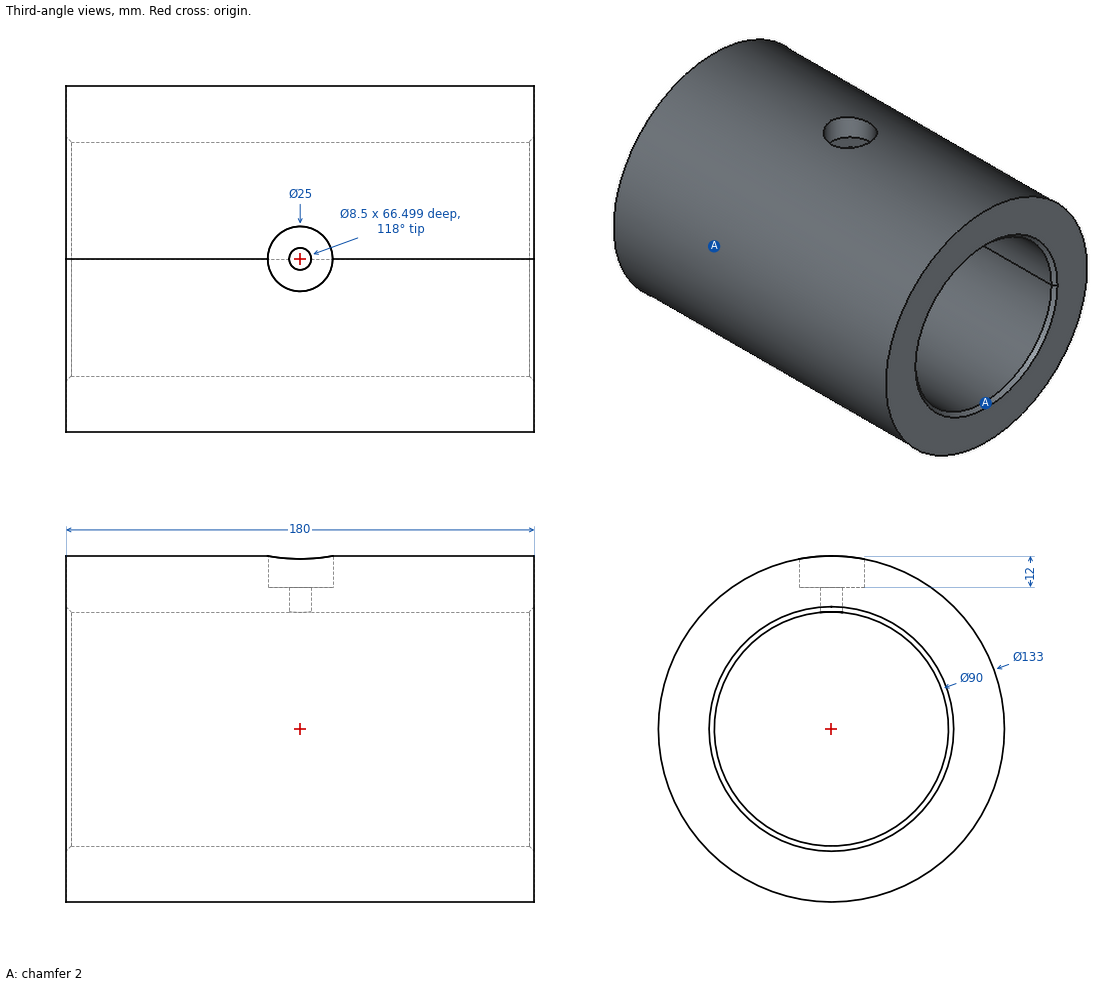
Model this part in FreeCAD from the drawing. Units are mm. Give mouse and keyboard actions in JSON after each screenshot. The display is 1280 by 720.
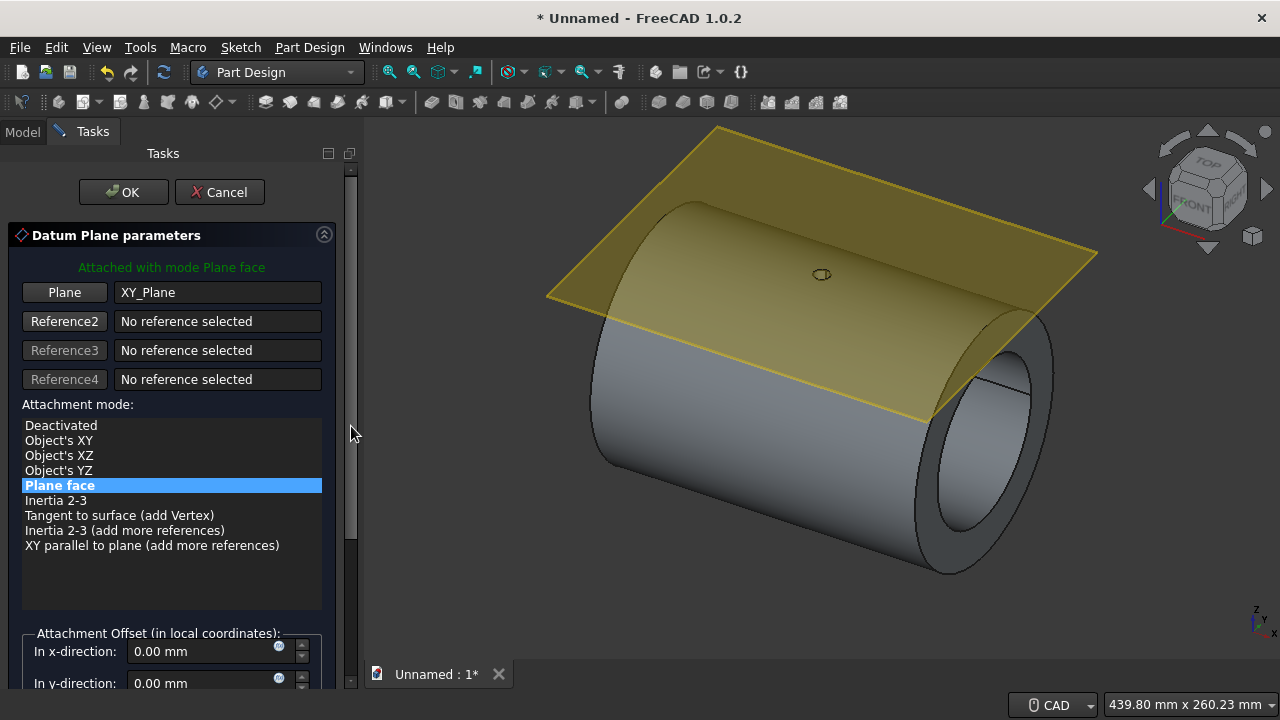
{"action": "left_click", "coordinate": [124, 192]}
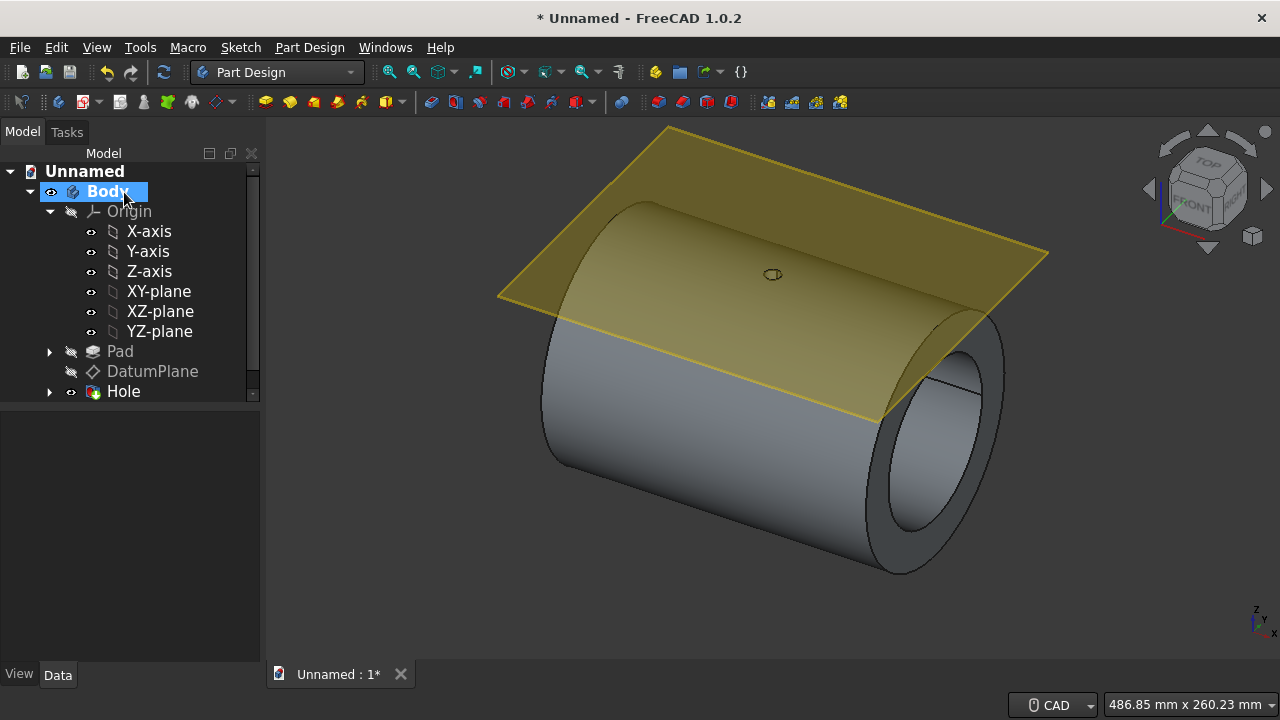
{"action": "scroll", "coordinate": [100, 287], "scroll_direction": "down", "scroll_amount": 3}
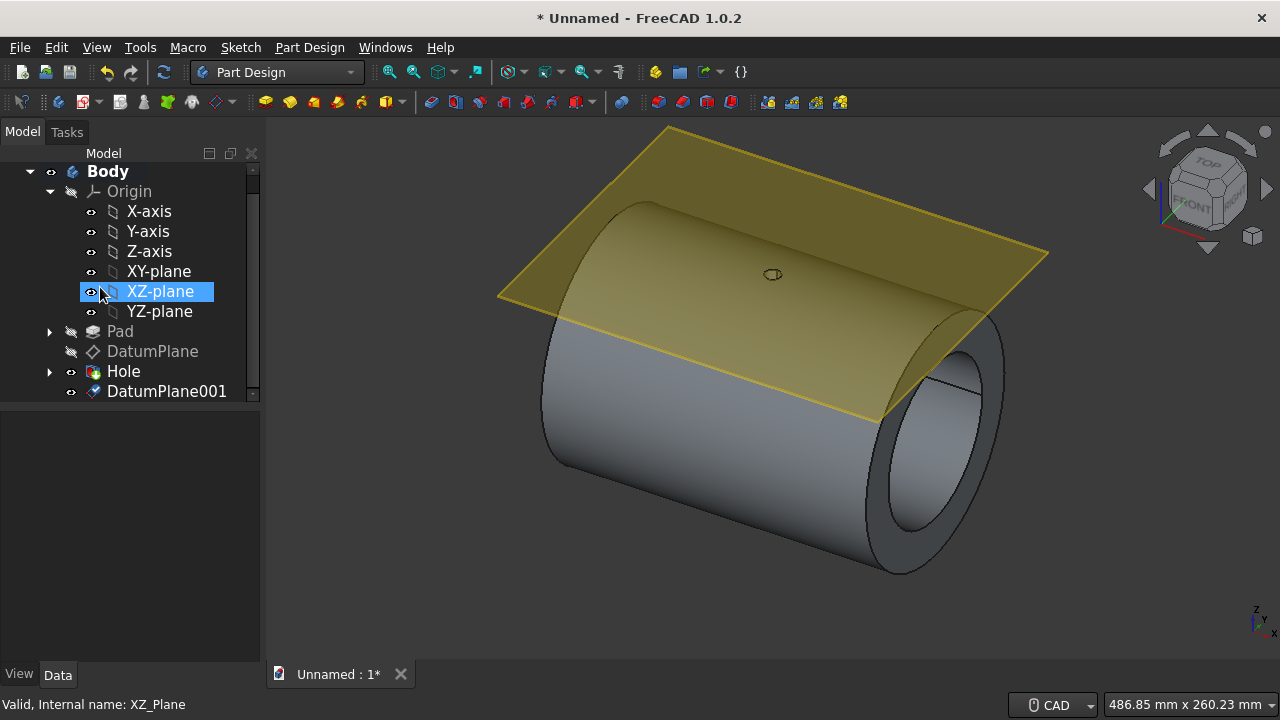
{"action": "left_click", "coordinate": [116, 392]}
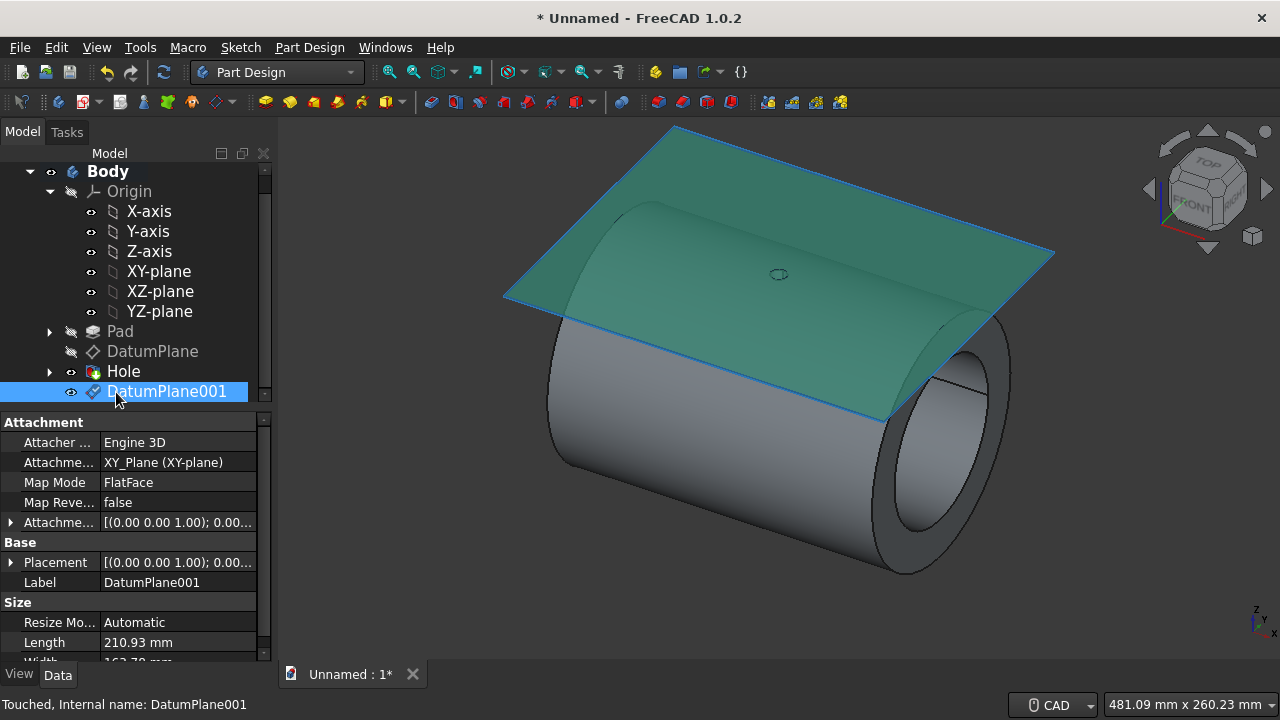
{"action": "left_click", "coordinate": [84, 102]}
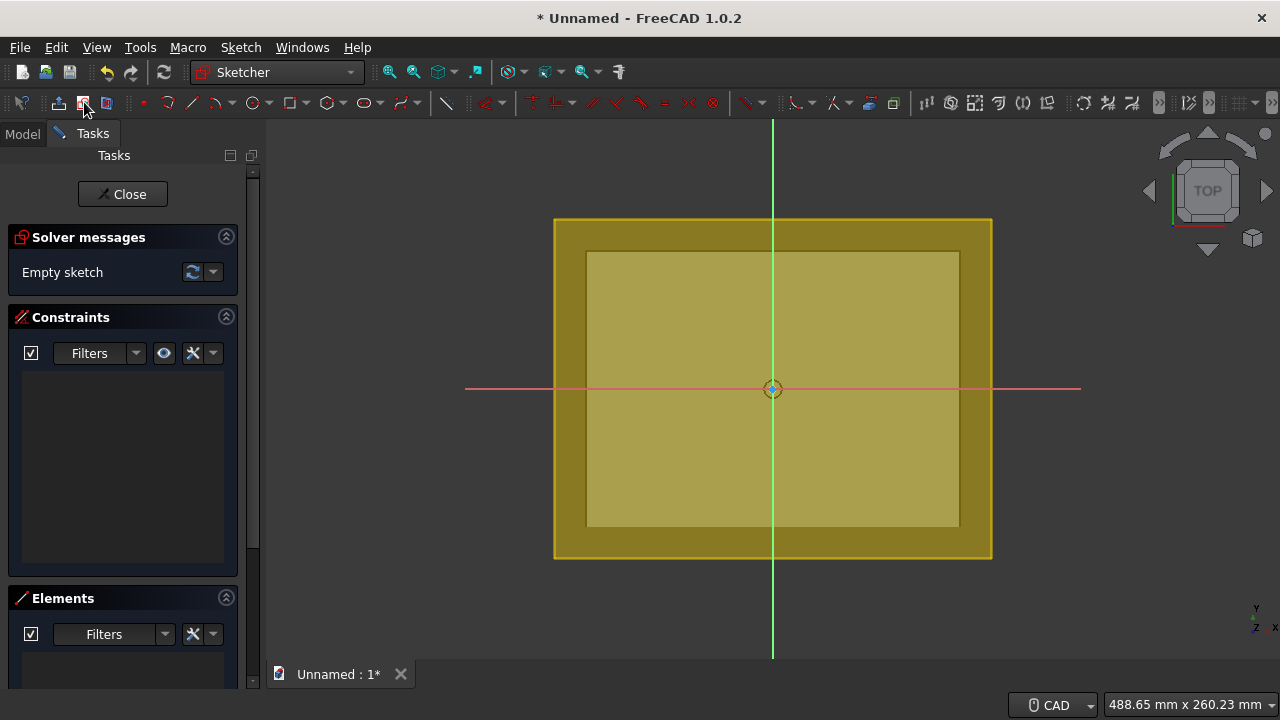
{"action": "scroll", "coordinate": [787, 389], "scroll_direction": "up", "scroll_amount": 9}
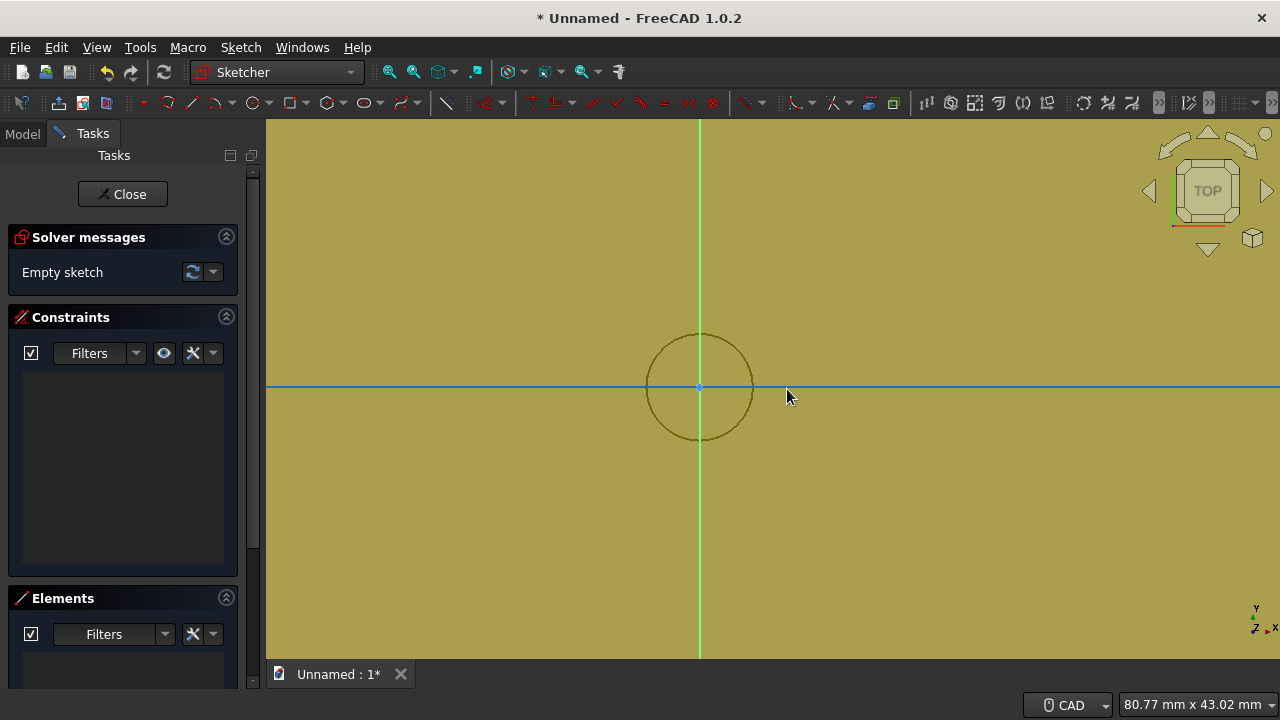
{"action": "left_click", "coordinate": [254, 104]}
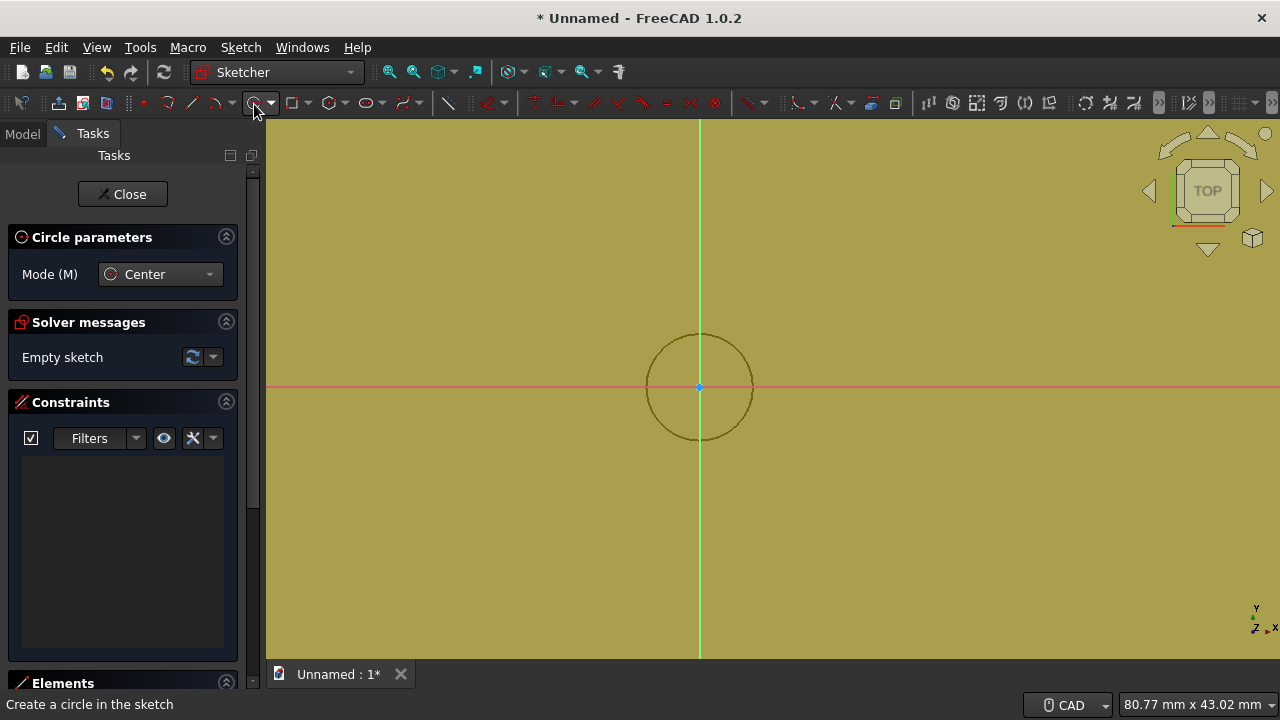
{"action": "left_click", "coordinate": [700, 387]}
{"action": "mouse_move", "coordinate": [811, 276]}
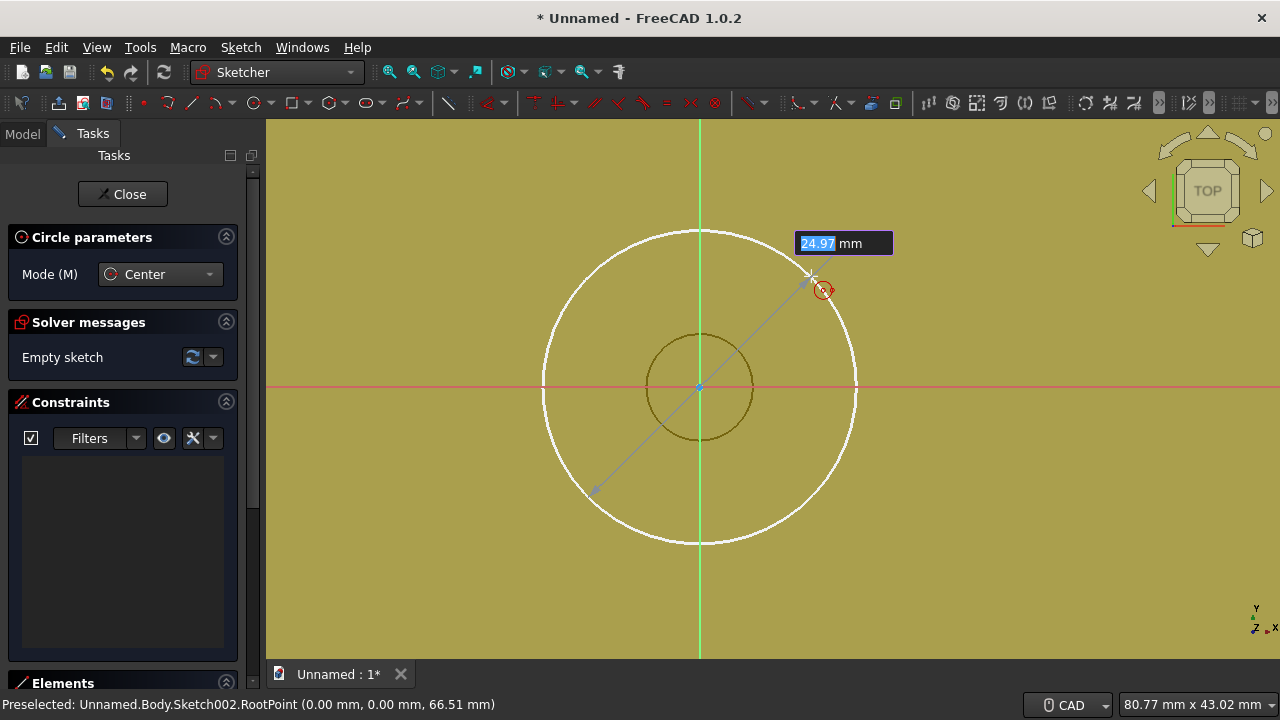
{"action": "type", "text": "25"}
{"action": "key", "text": "Return"}
{"action": "key", "text": "Escape"}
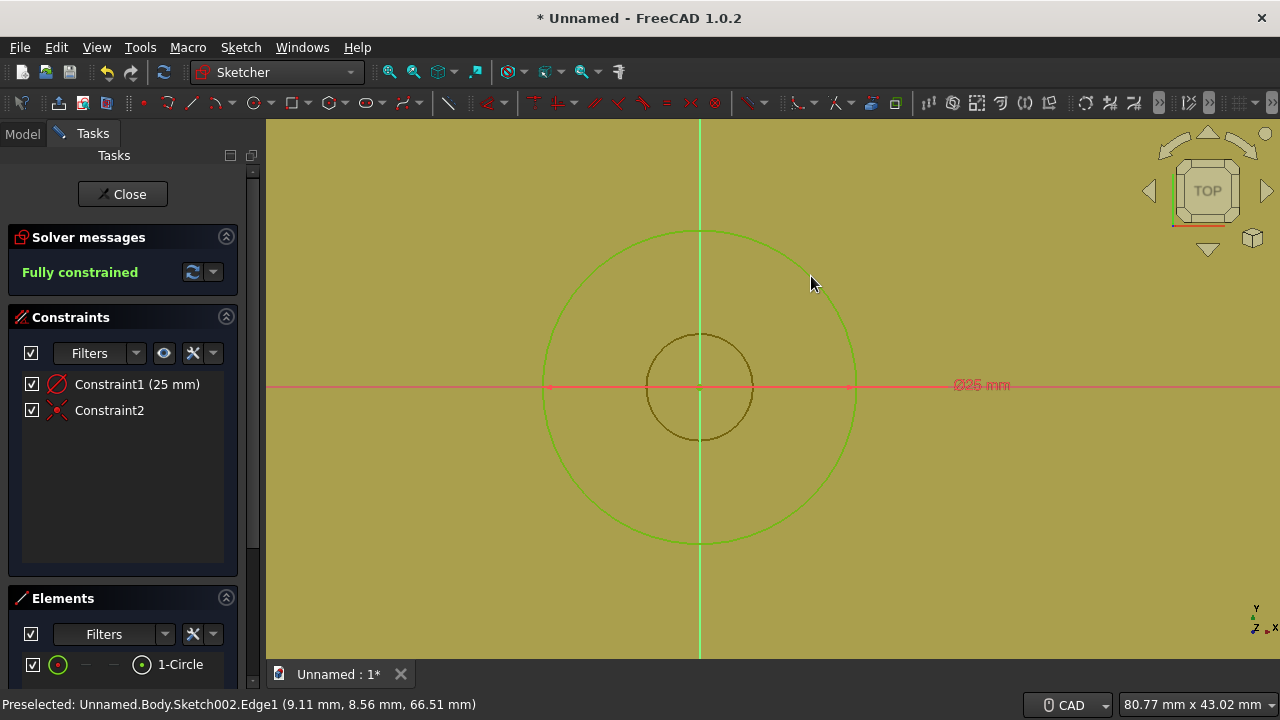
{"action": "left_click", "coordinate": [123, 194]}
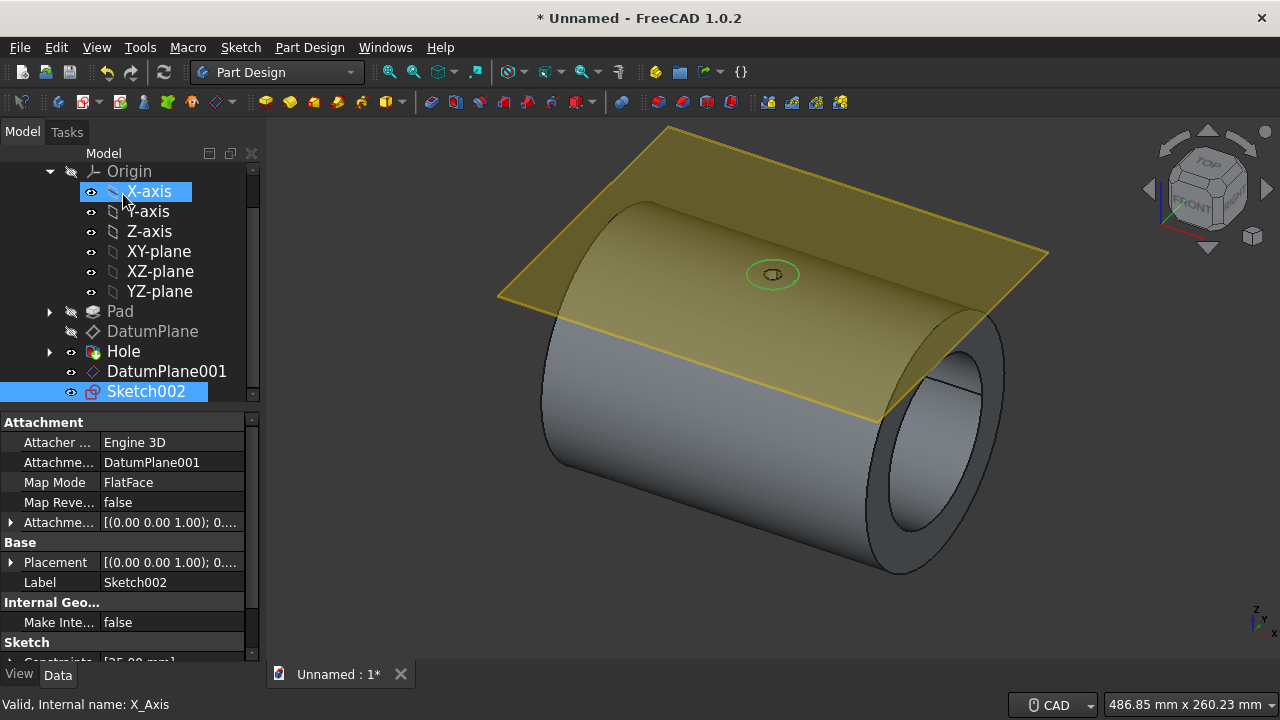
{"action": "left_click", "coordinate": [432, 102]}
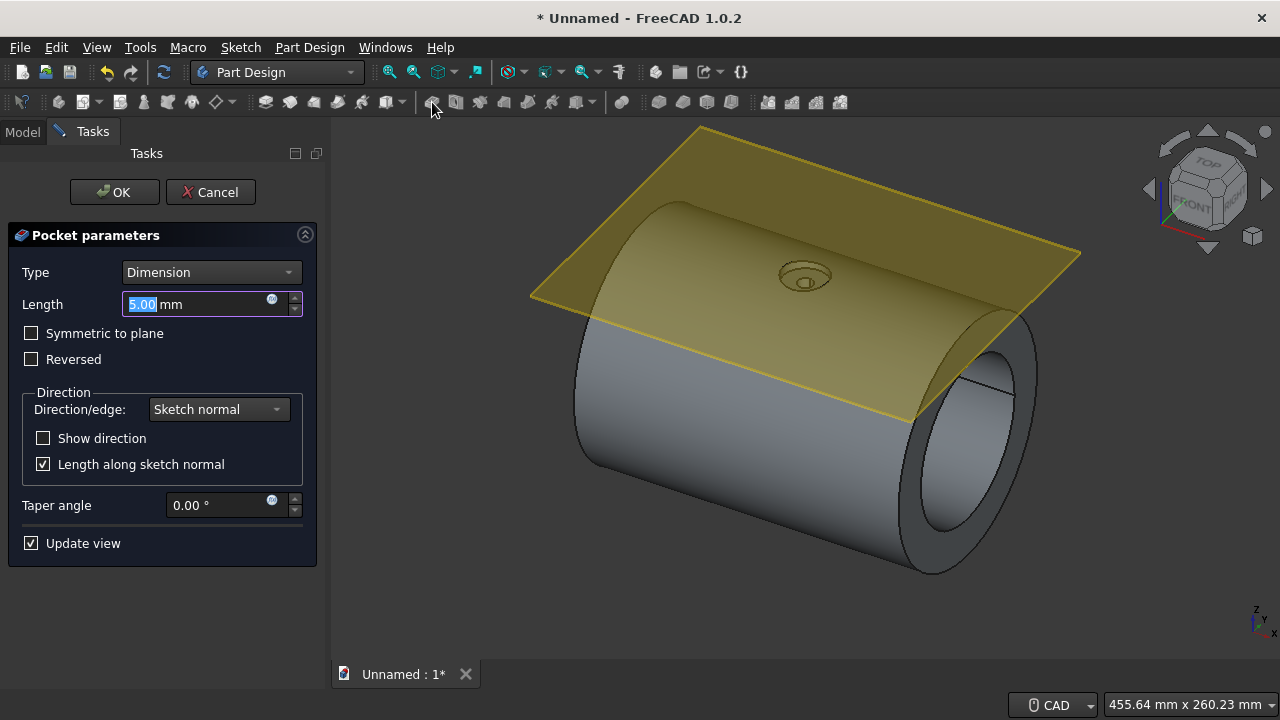
{"action": "type", "text": "12"}
{"action": "key", "text": "Tab"}